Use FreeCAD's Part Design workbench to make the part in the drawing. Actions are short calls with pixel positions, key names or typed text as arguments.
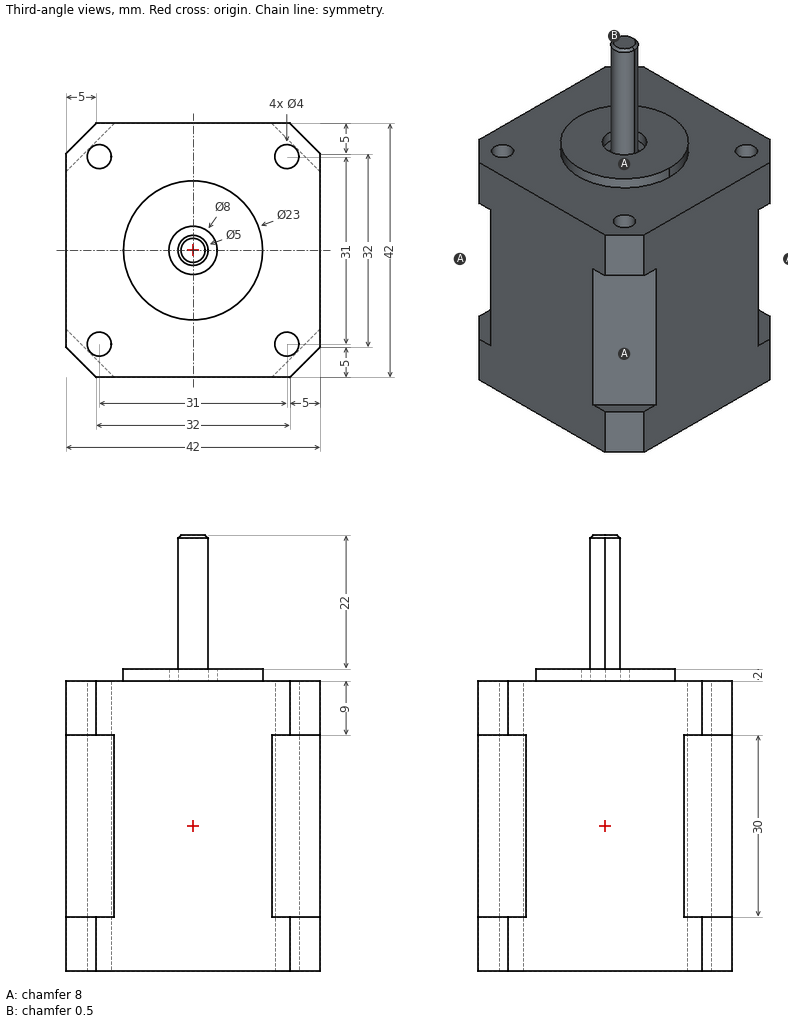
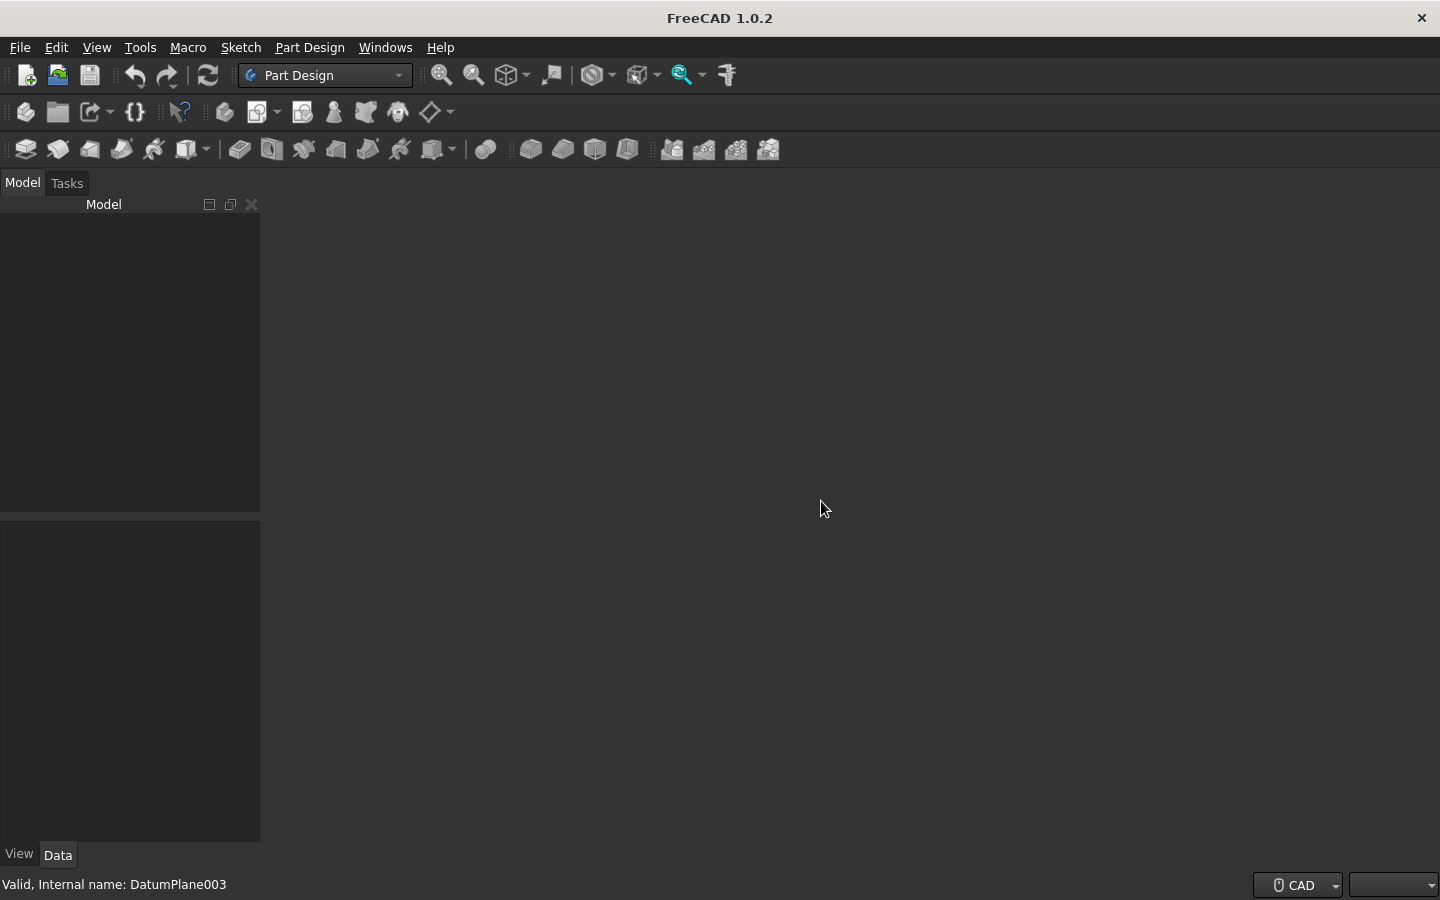
click(26, 76)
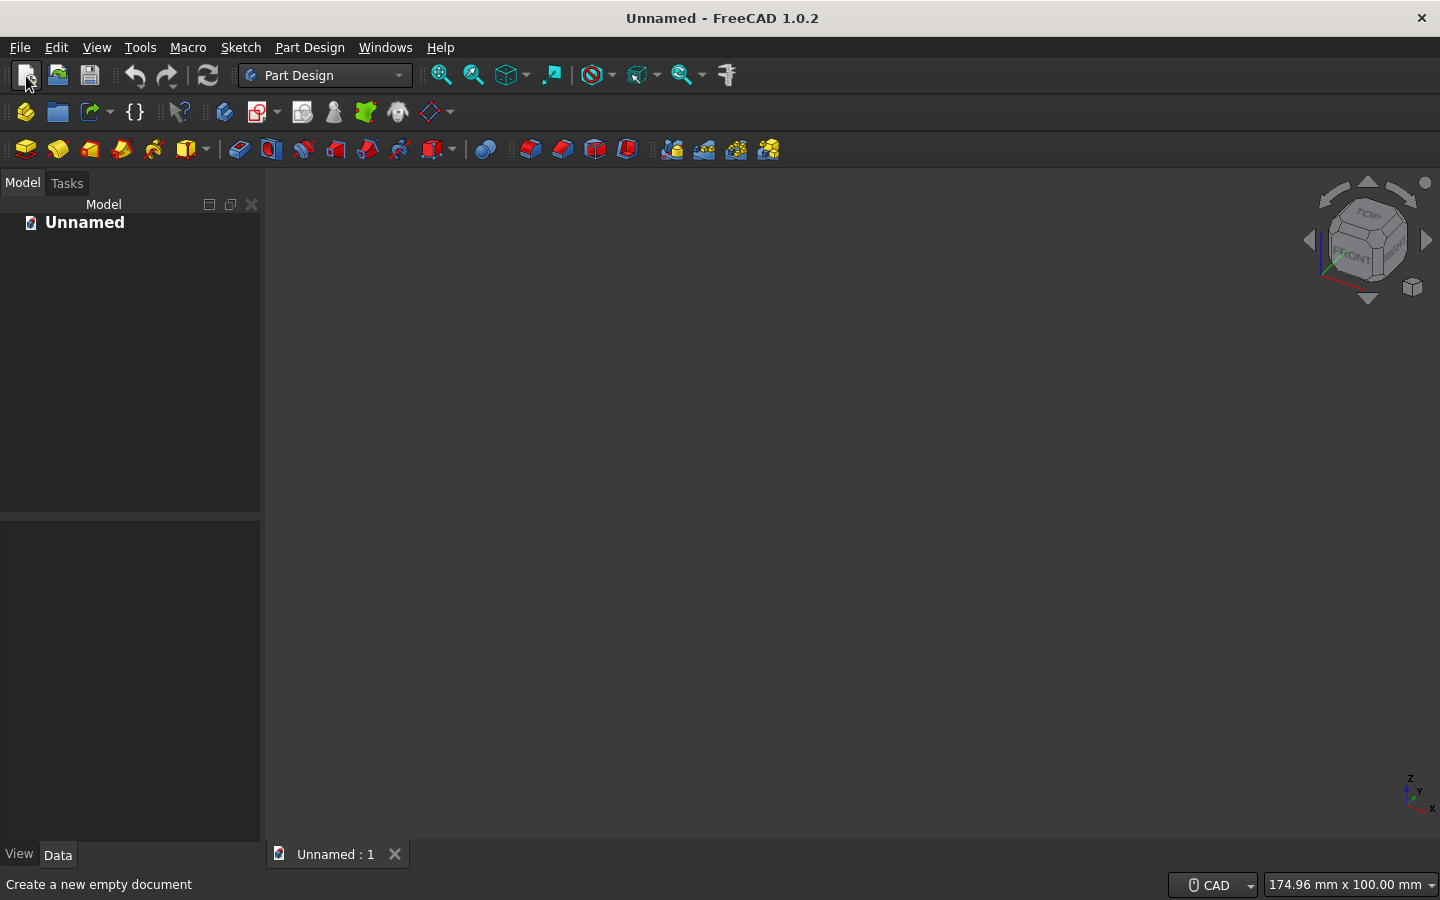
click(258, 112)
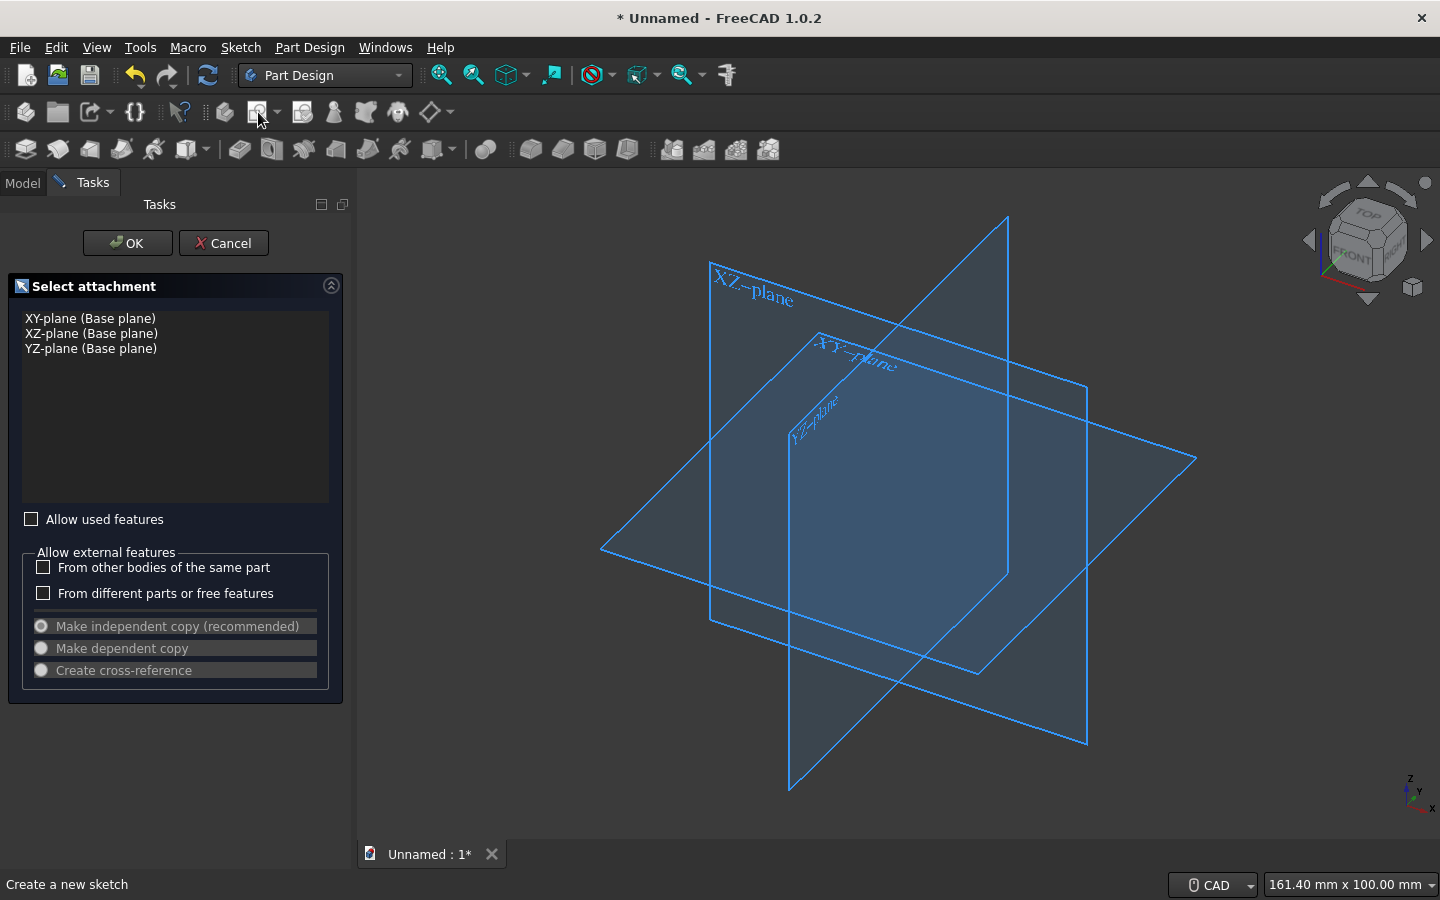
click(82, 318)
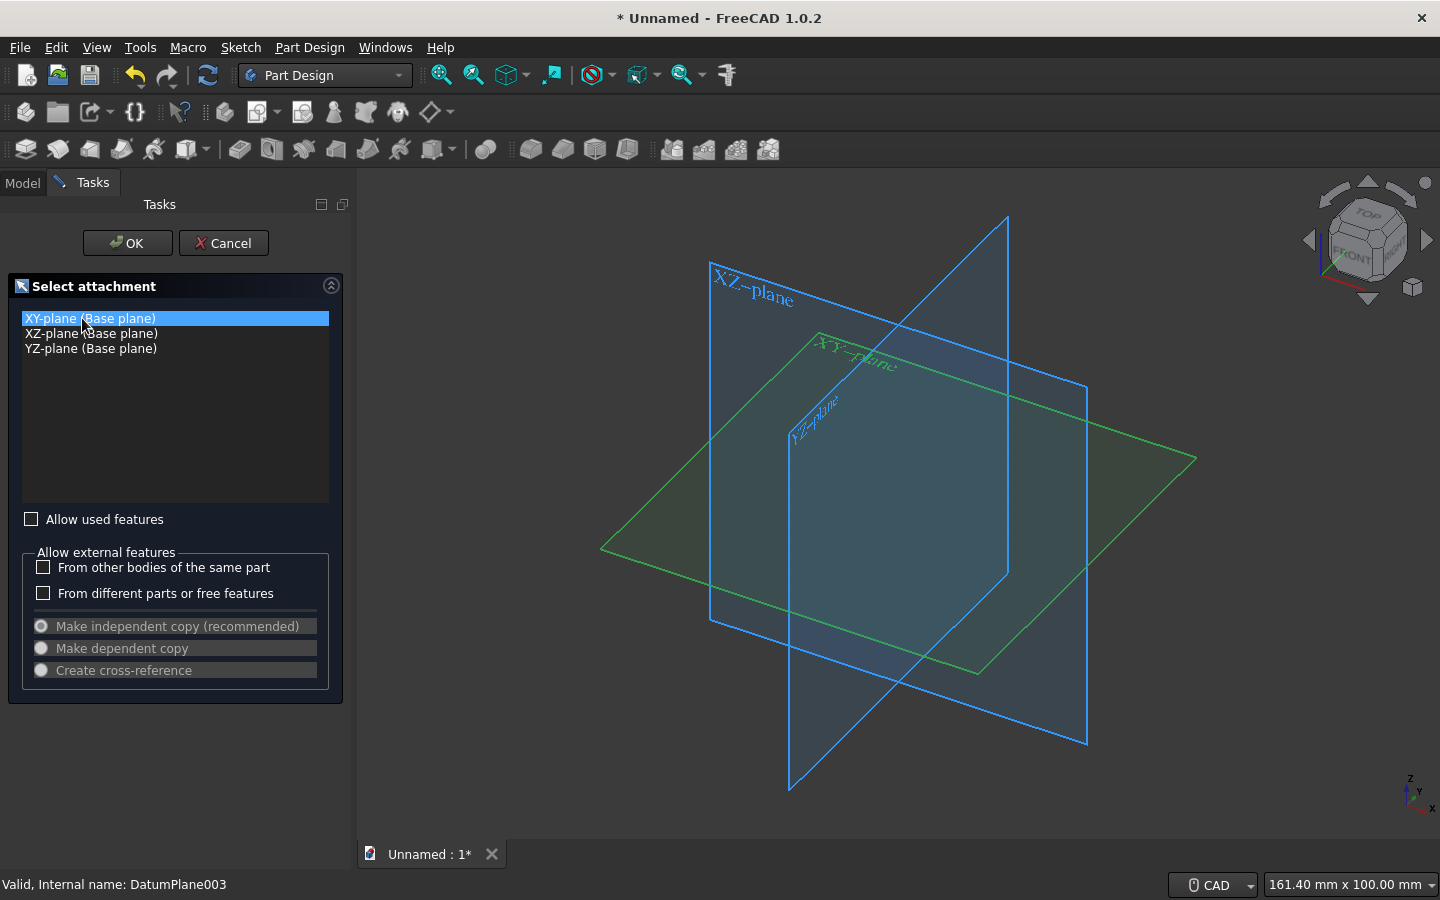
click(128, 243)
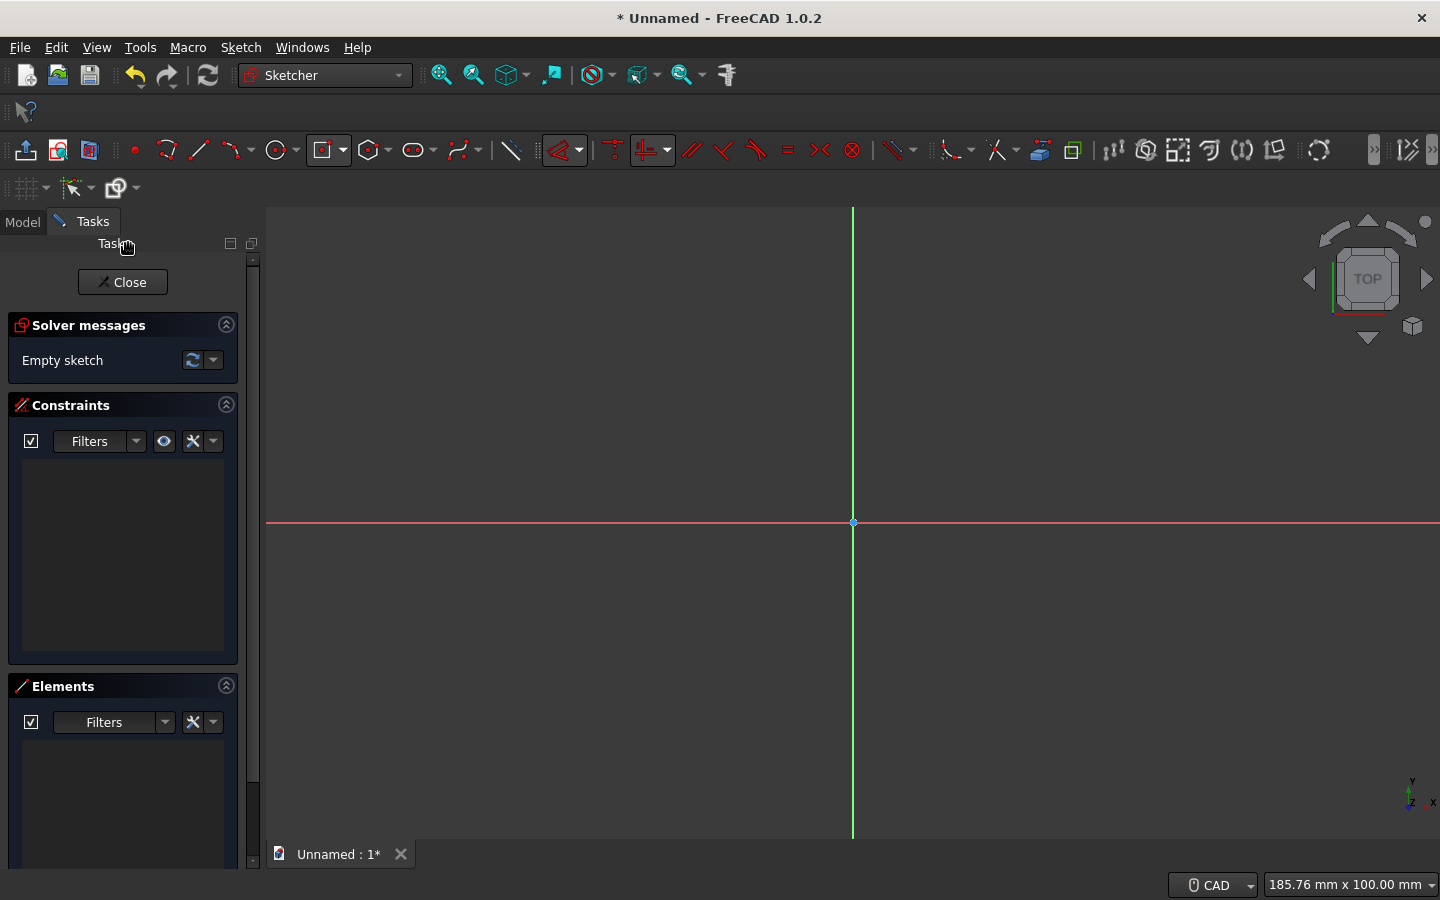
scroll(992, 523, up, 2)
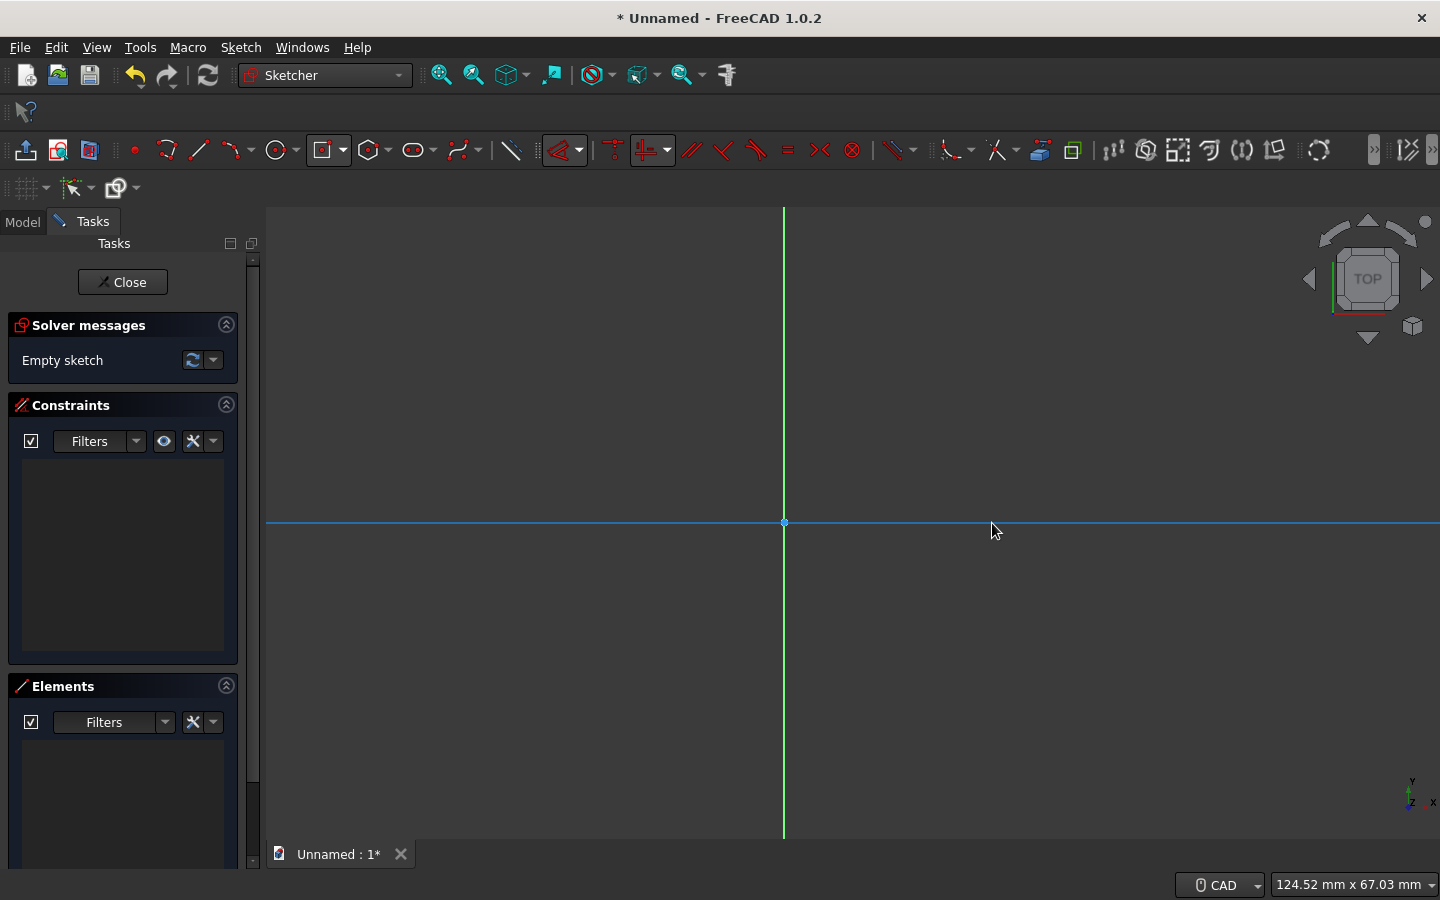
key(g)
key(v)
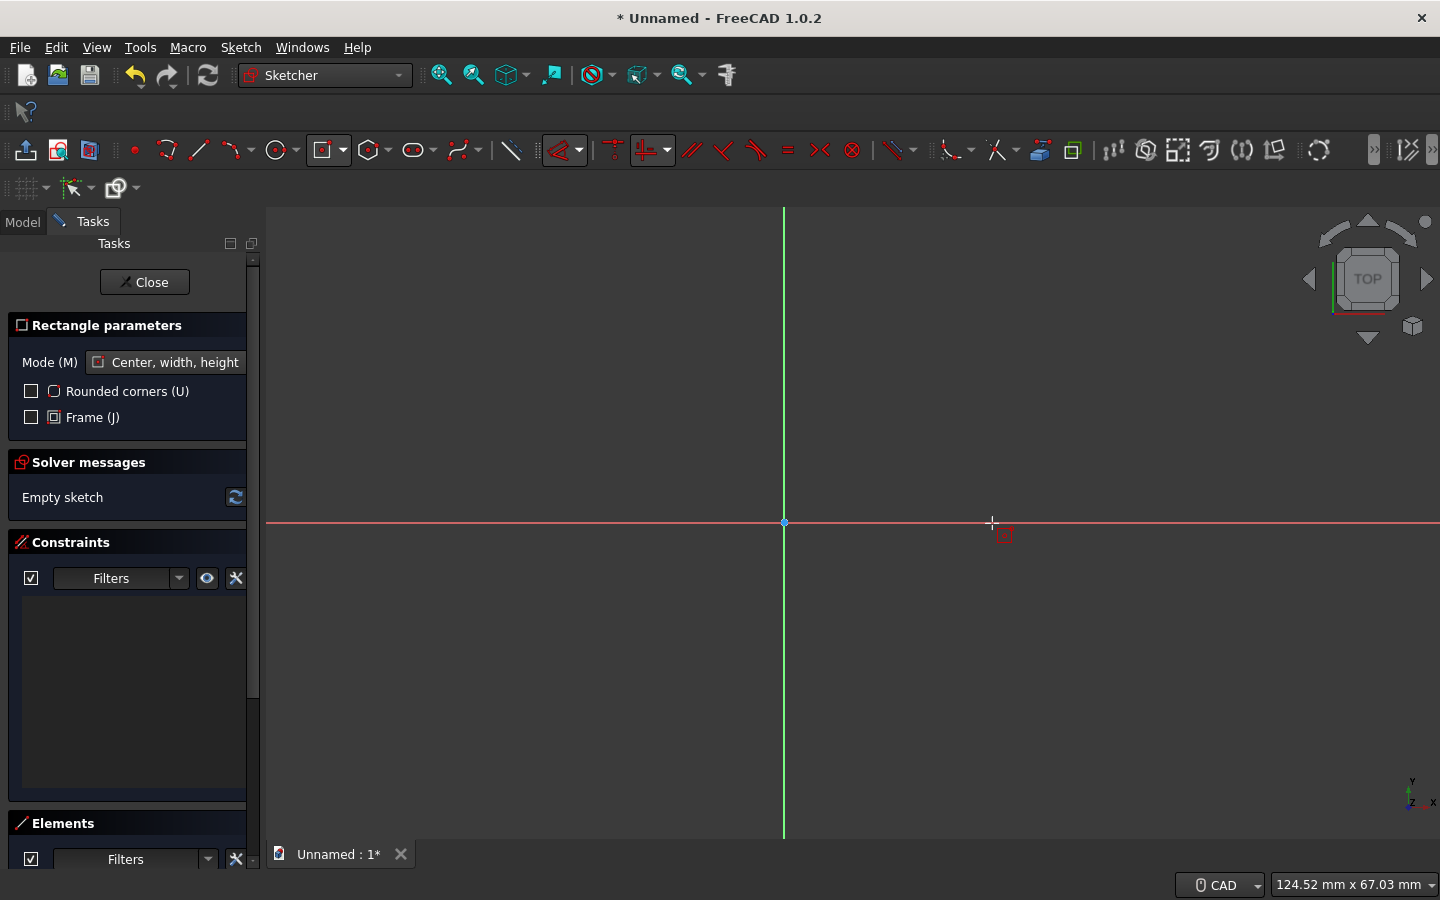
click(784, 523)
move(982, 325)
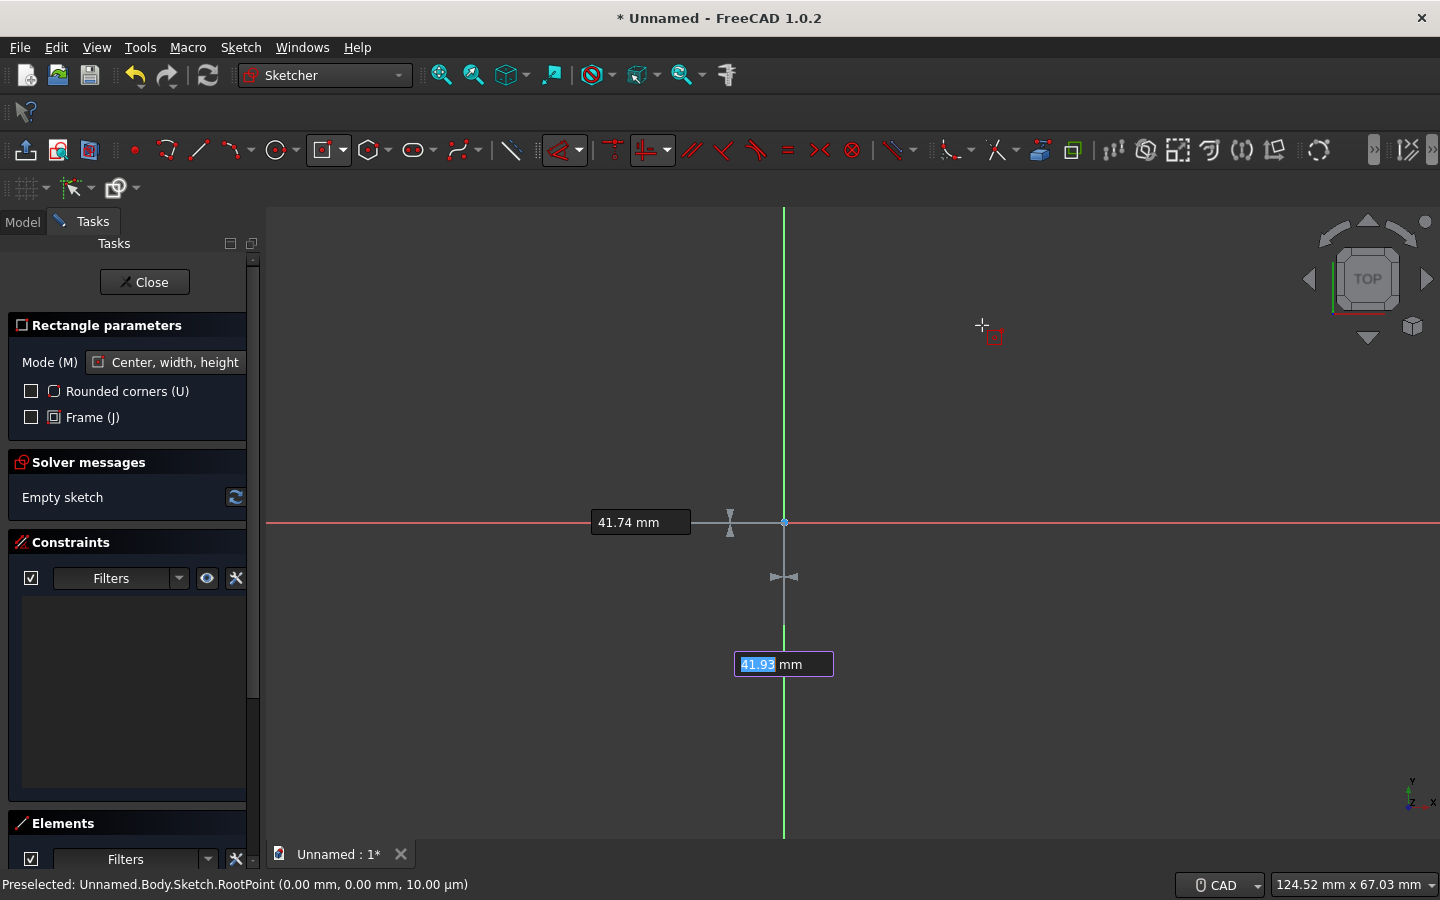
text(42)
key(Tab)
text(42)
key(Return)
key(Escape)